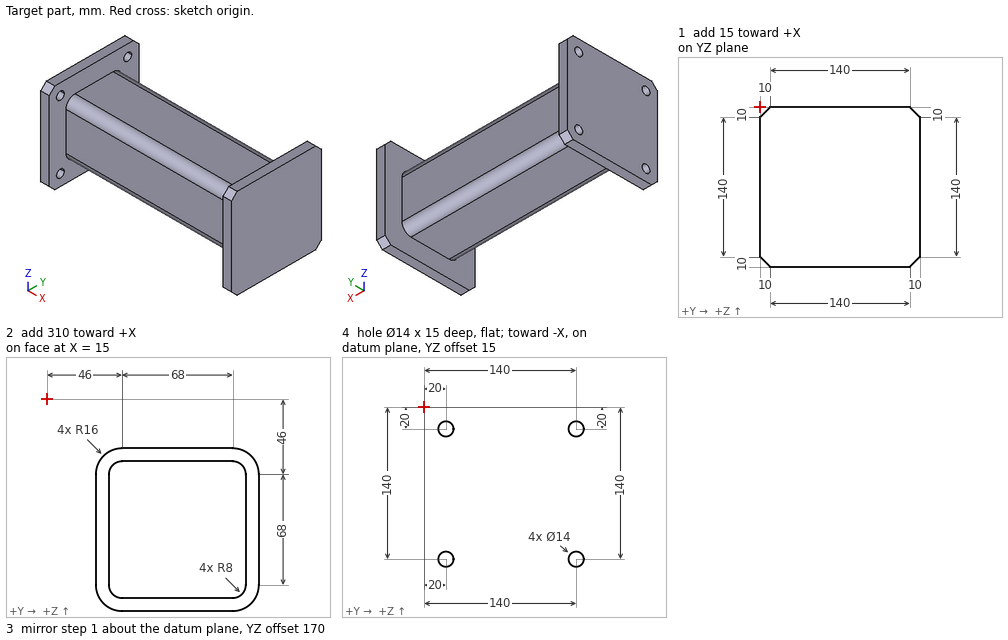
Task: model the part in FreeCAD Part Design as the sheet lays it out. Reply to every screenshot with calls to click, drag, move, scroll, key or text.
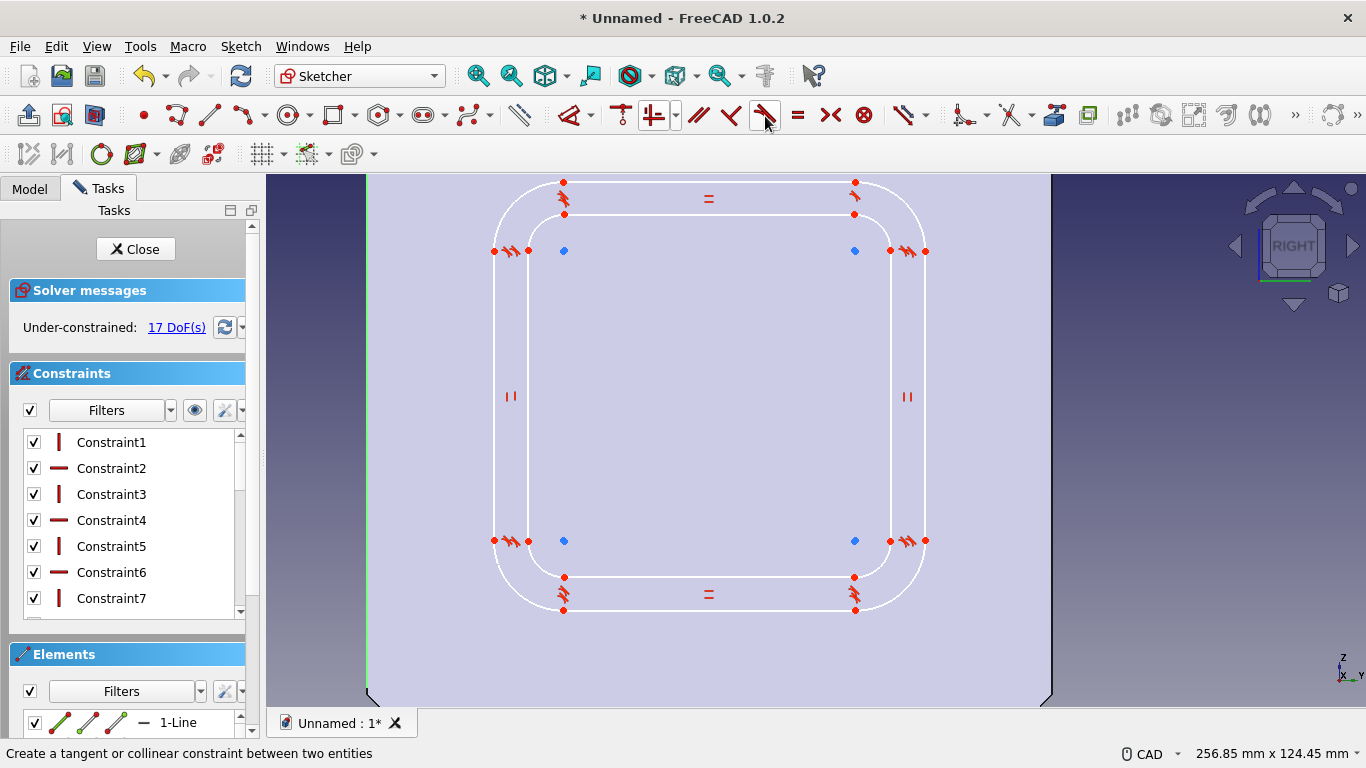
click(651, 215)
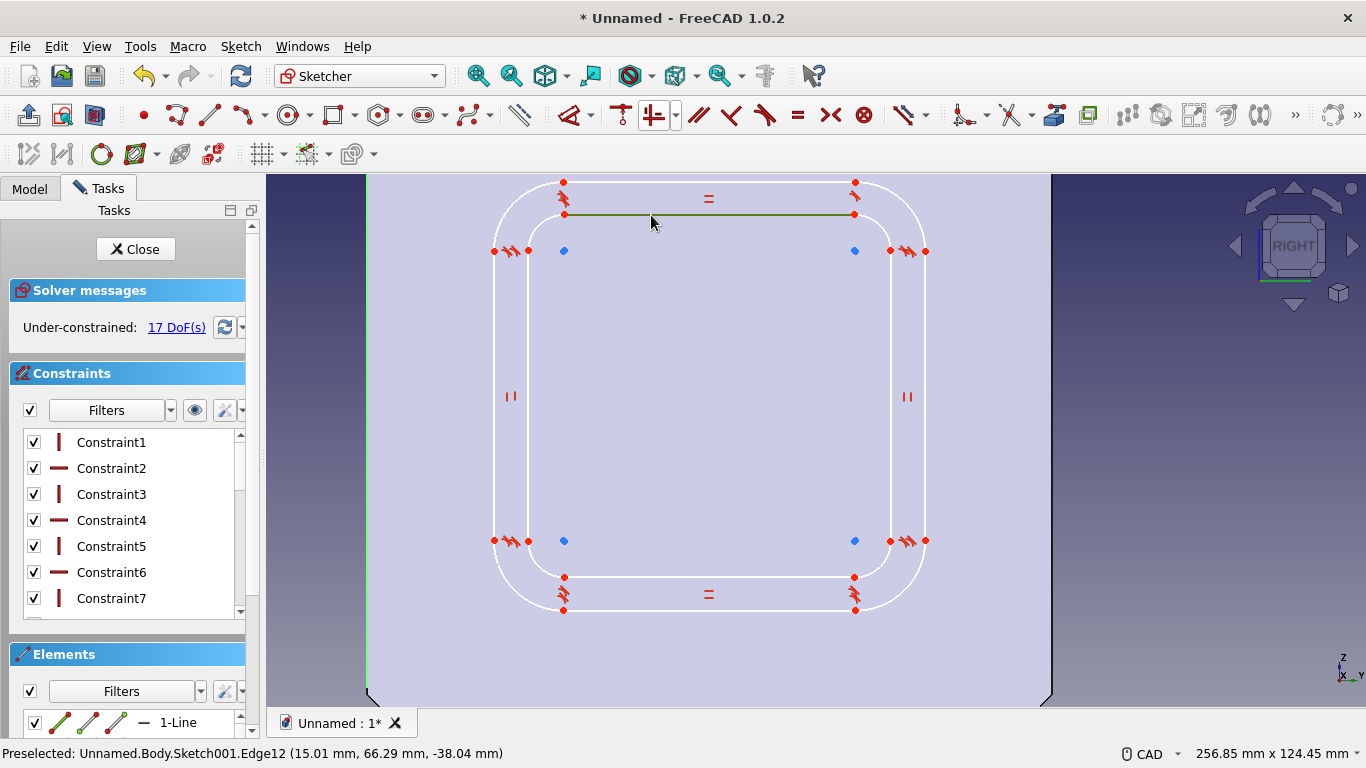
click(887, 235)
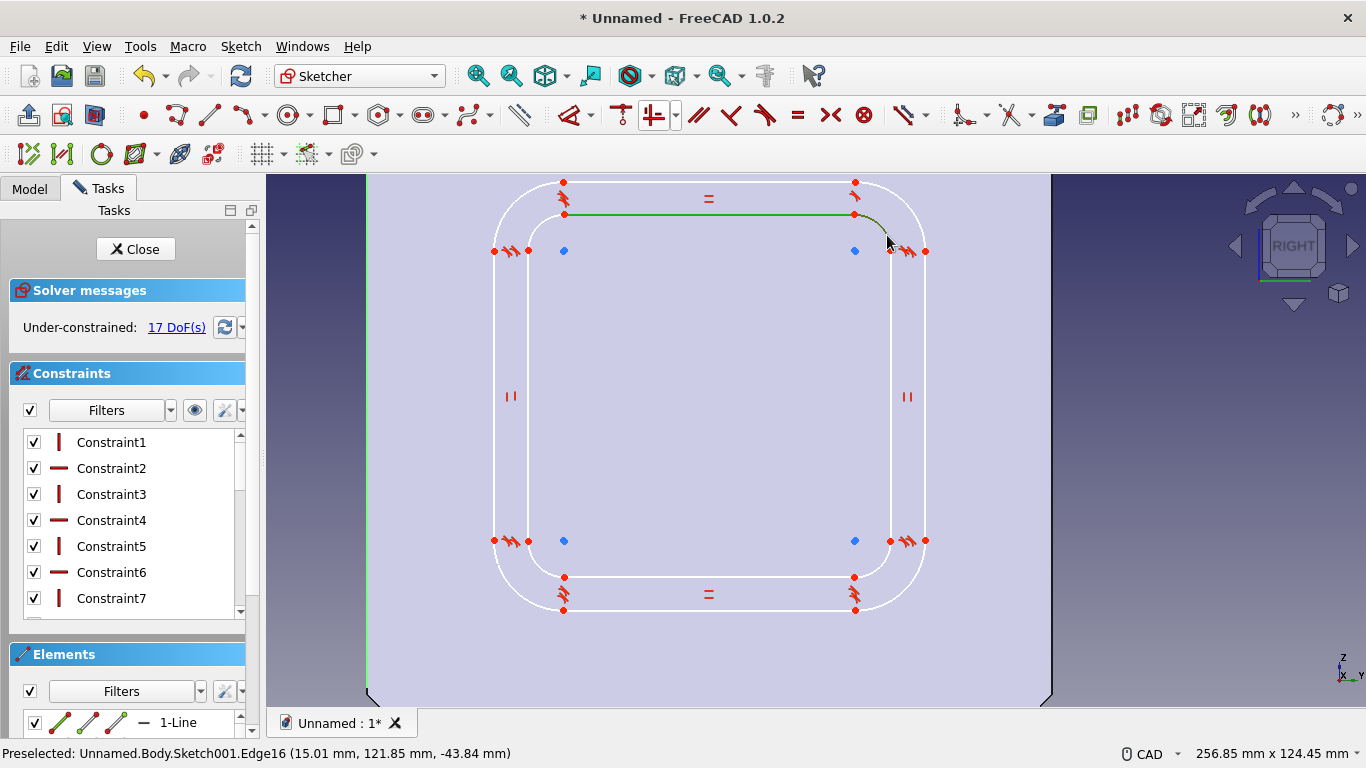
key(t)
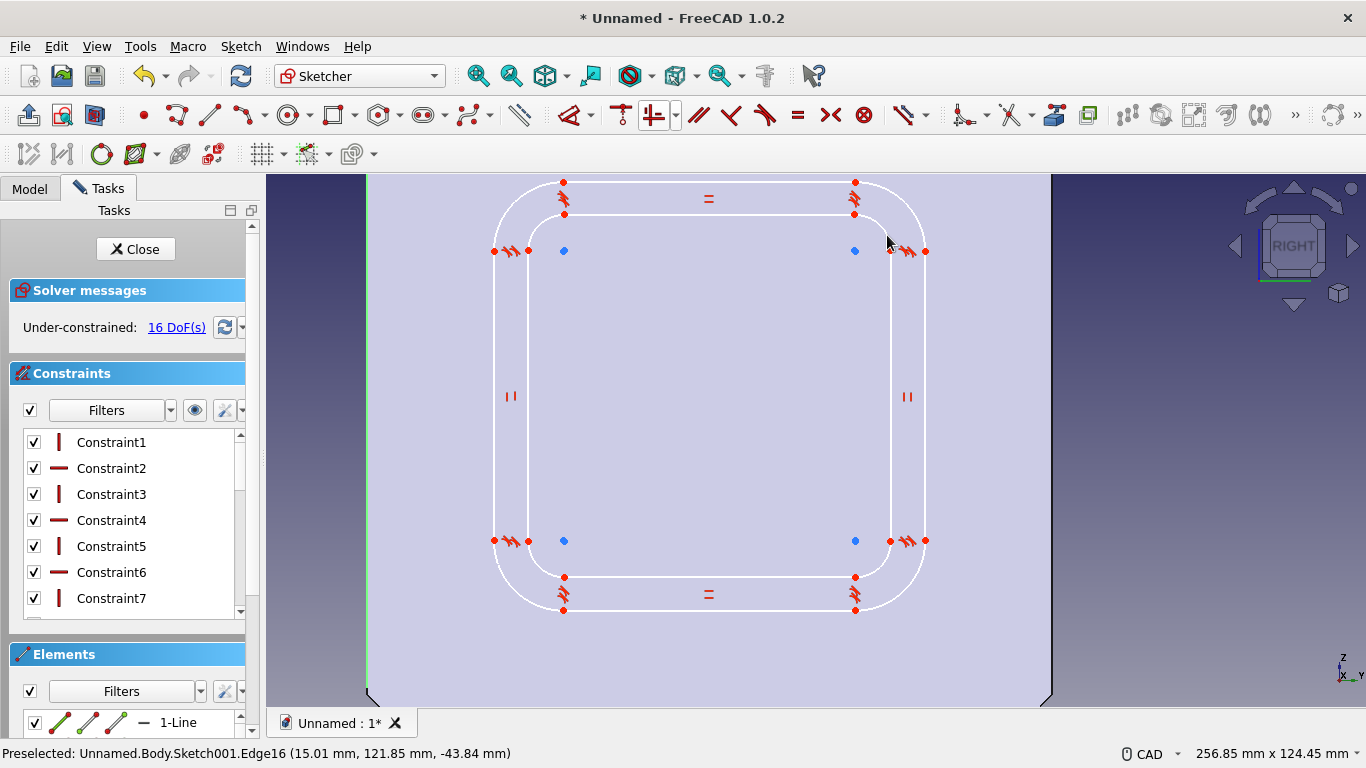
click(887, 603)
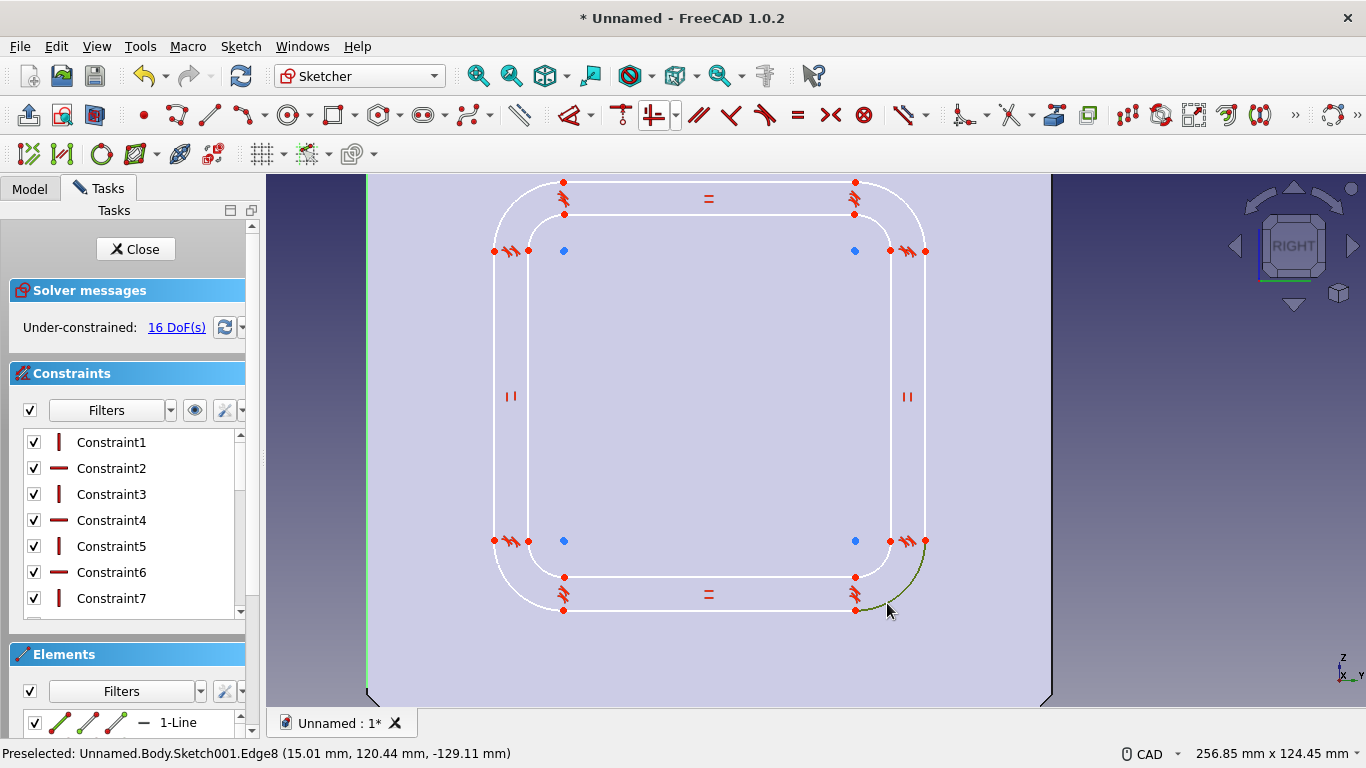
click(871, 573)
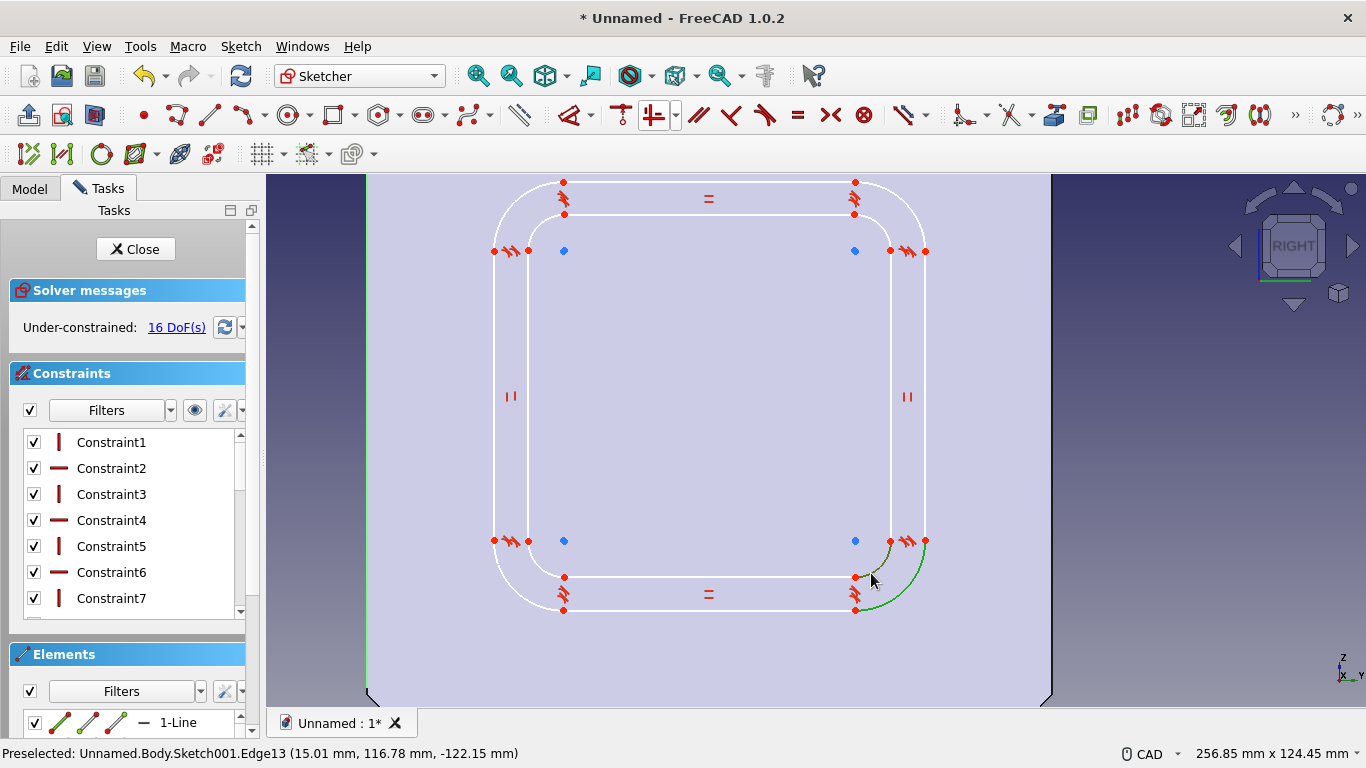
key(c)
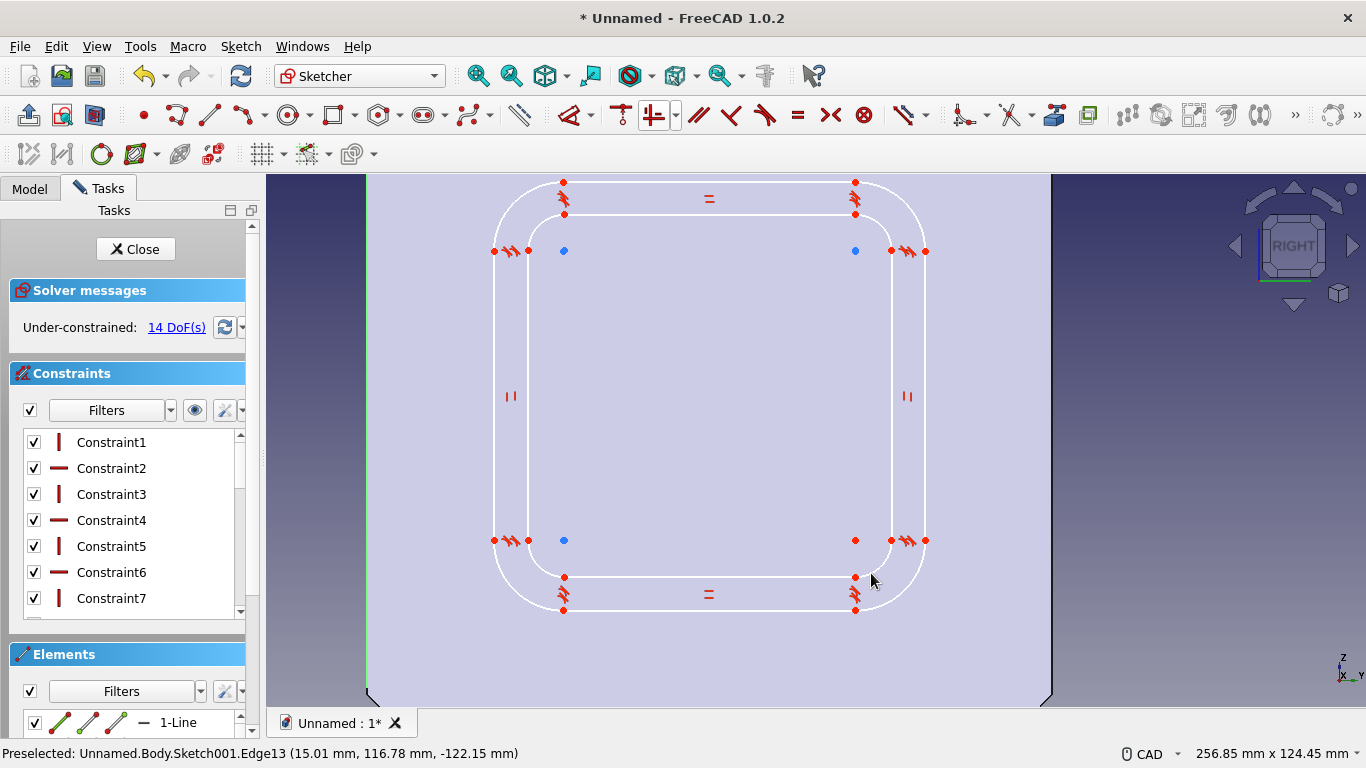
click(502, 573)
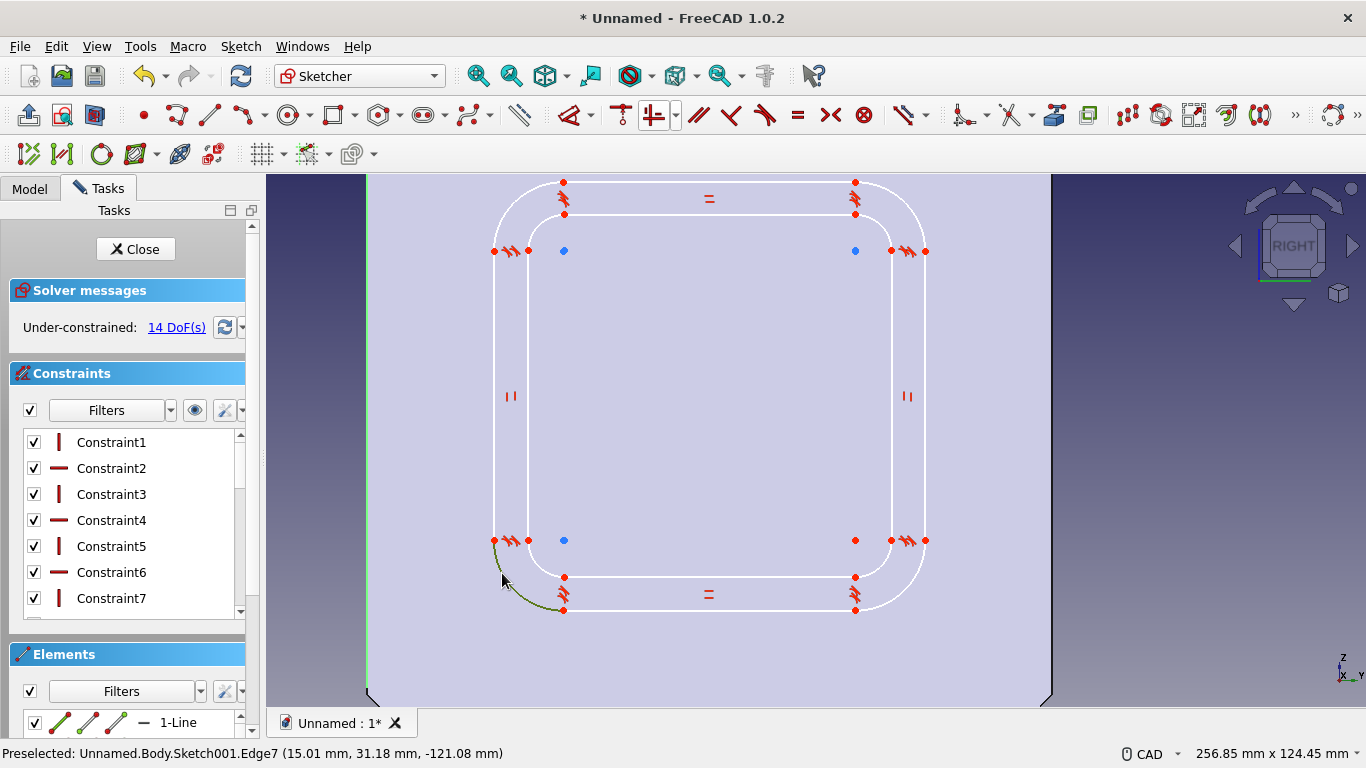
click(532, 557)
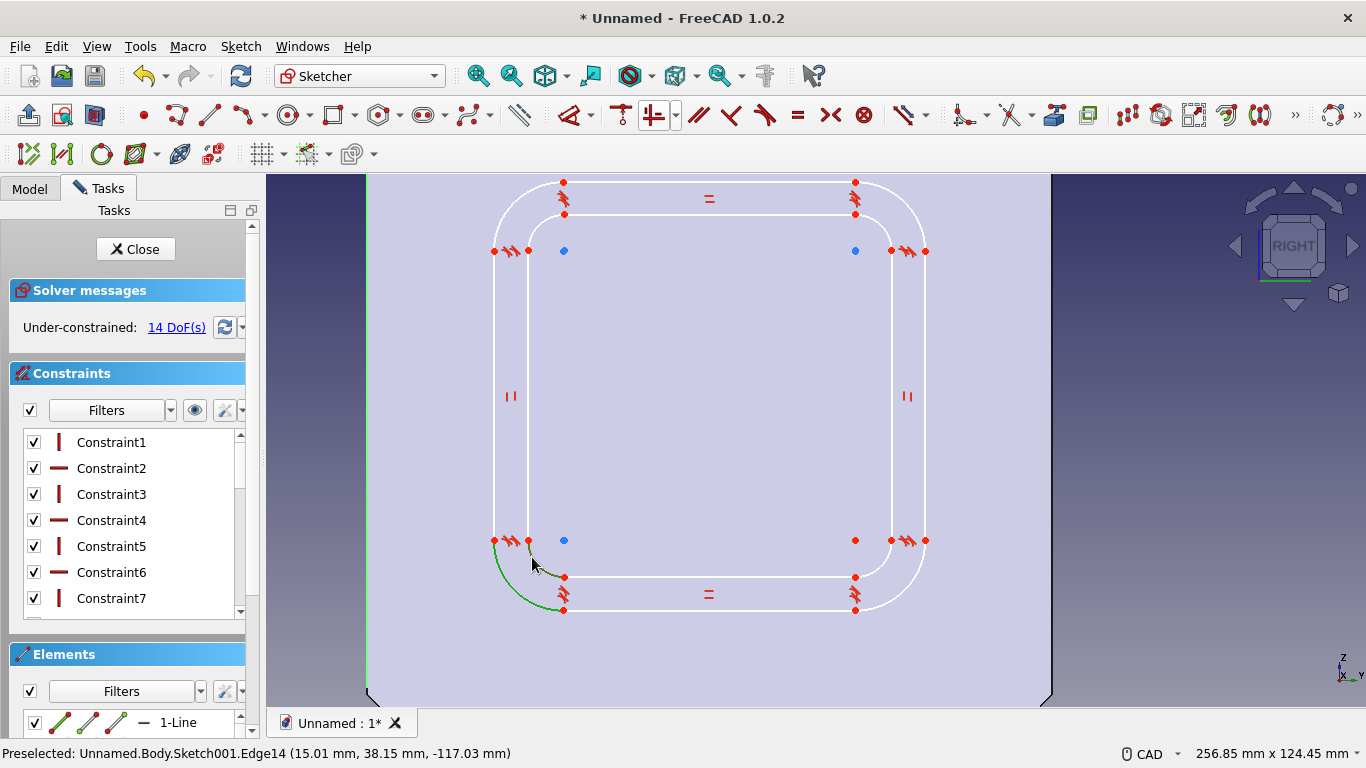
key(c)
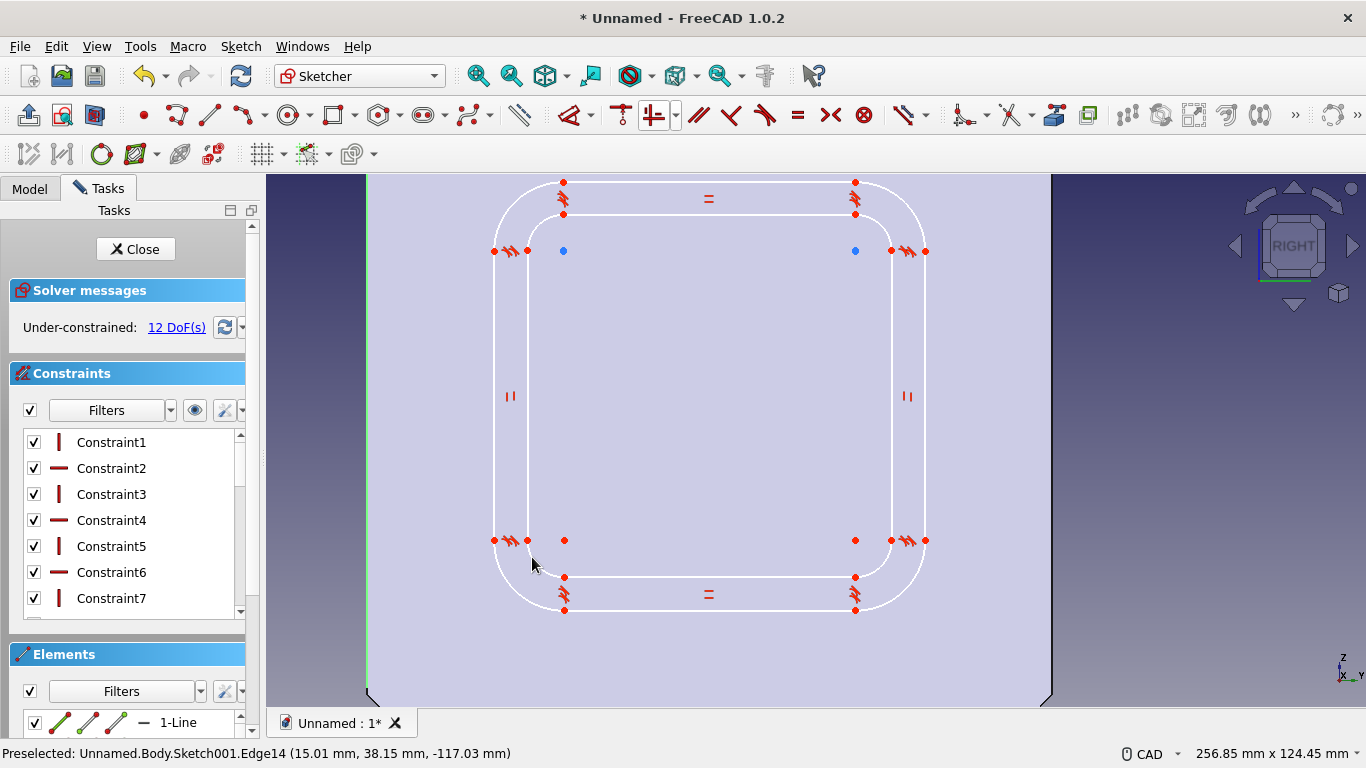
click(502, 220)